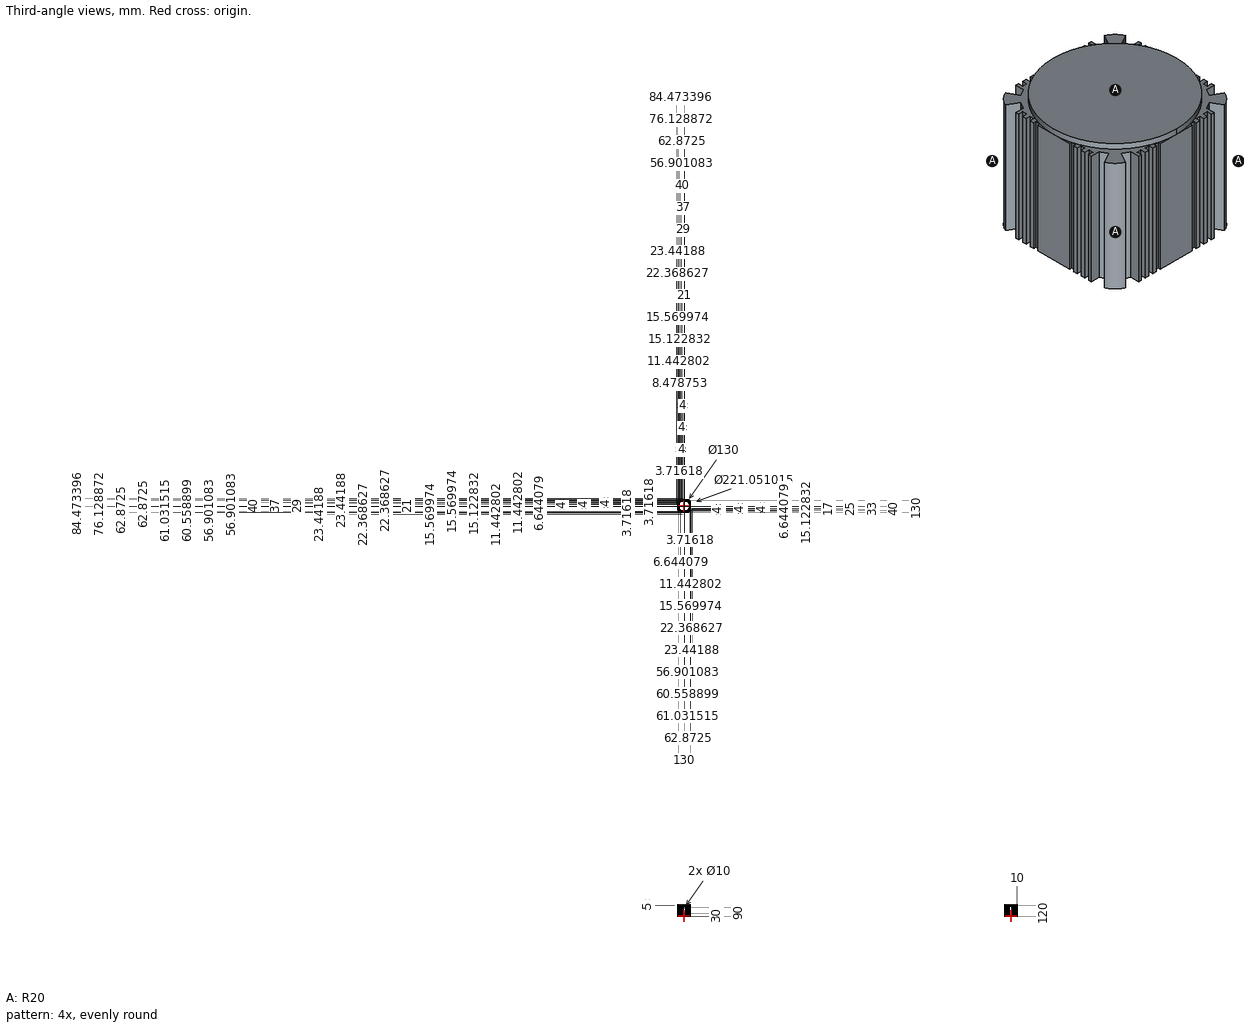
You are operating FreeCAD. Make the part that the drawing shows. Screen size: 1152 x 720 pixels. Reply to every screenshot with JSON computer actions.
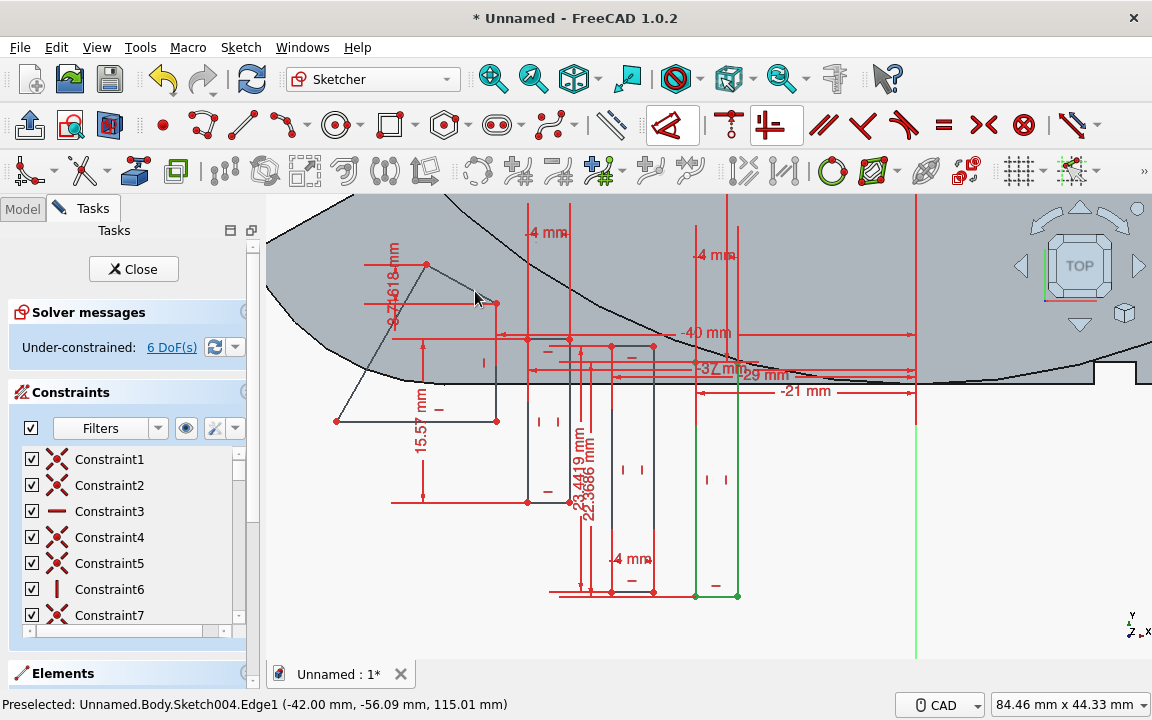
{"action": "left_click", "coordinate": [385, 422]}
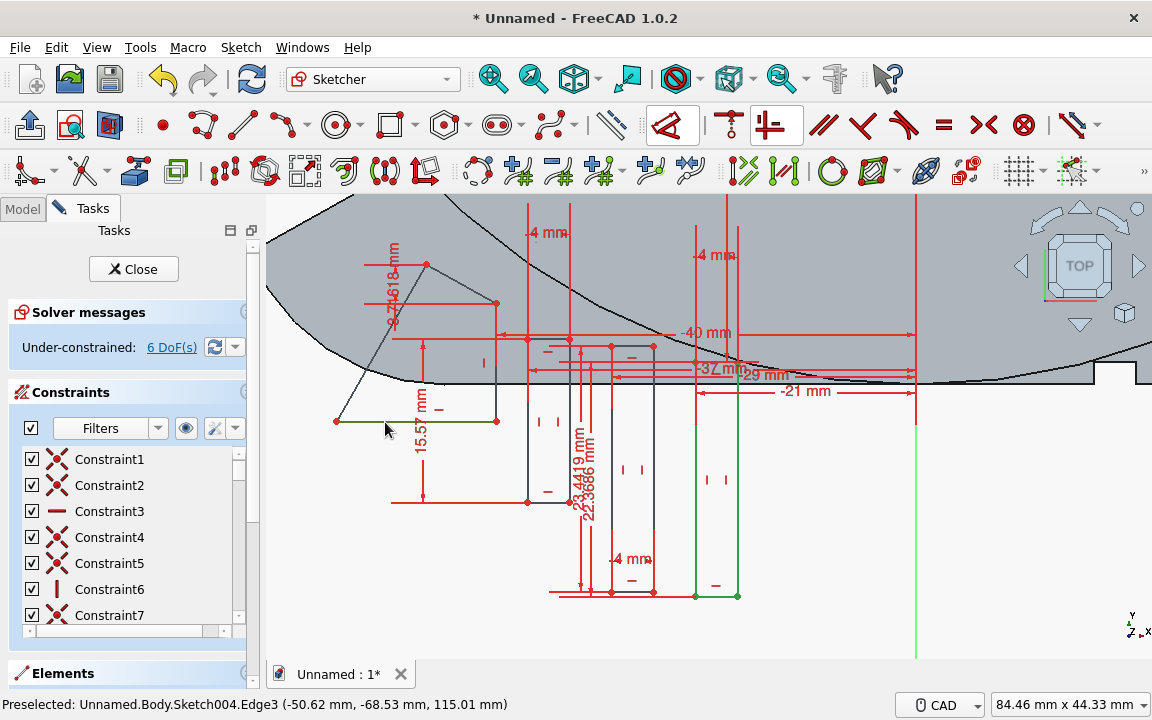
{"action": "left_click", "coordinate": [694, 126]}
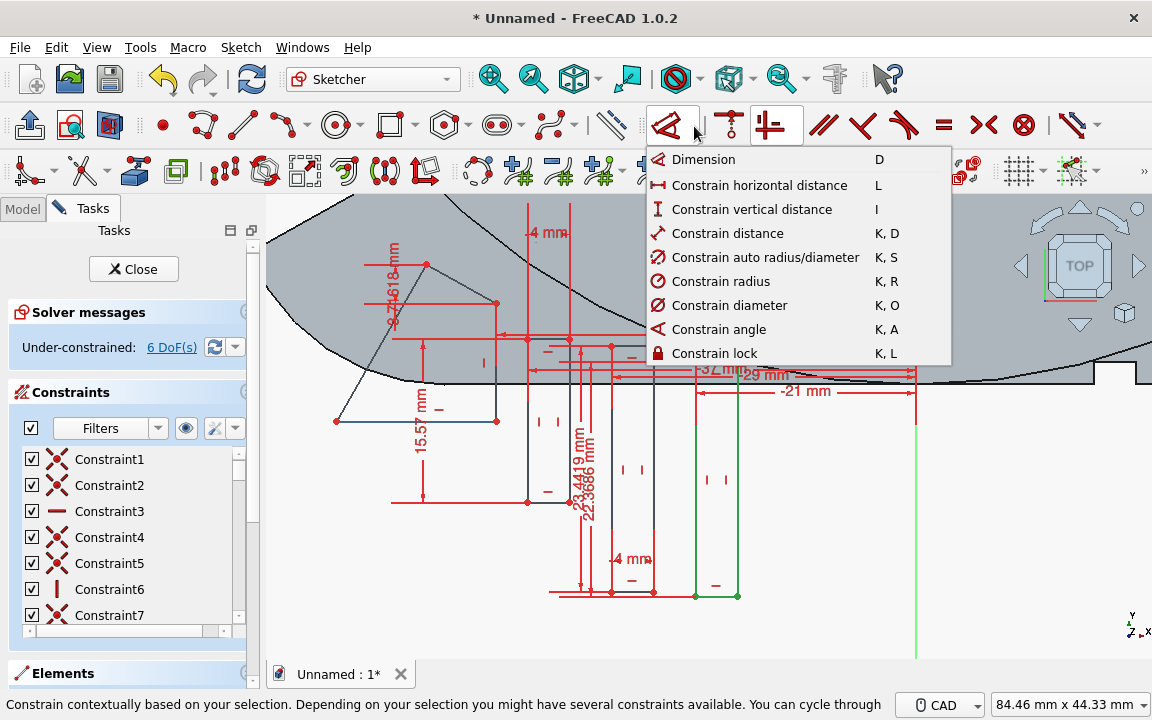
{"action": "left_click", "coordinate": [799, 185]}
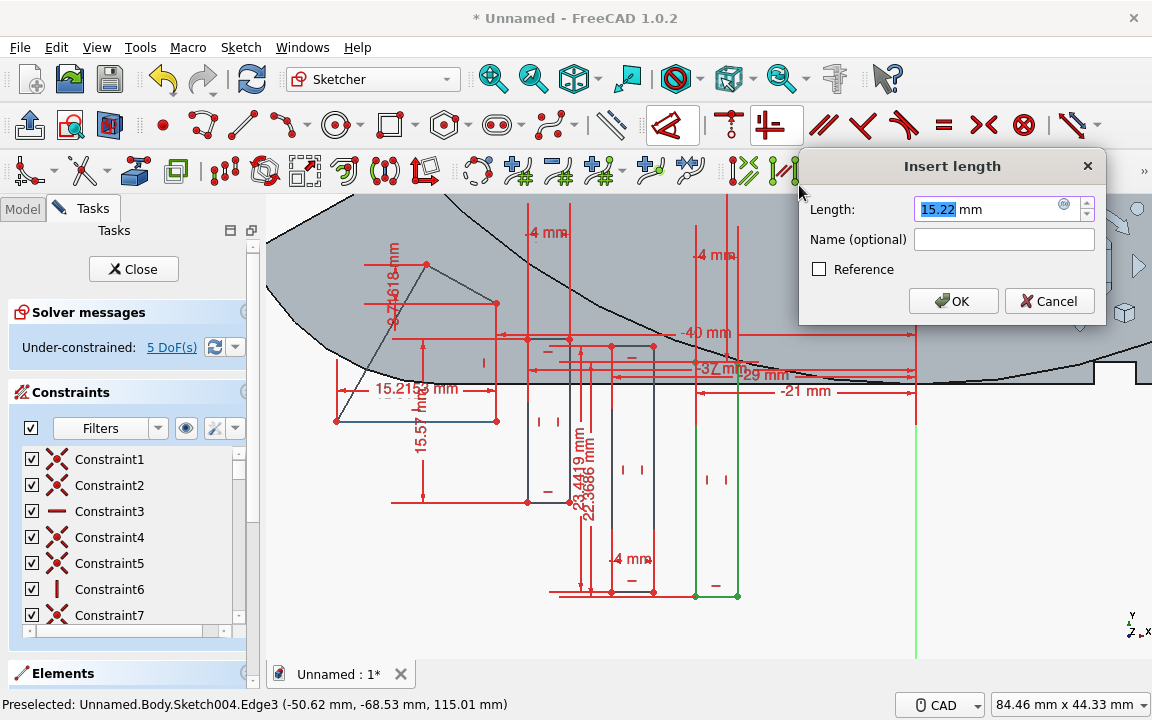
{"action": "type", "text": "15.122832"}
{"action": "key", "text": "Return"}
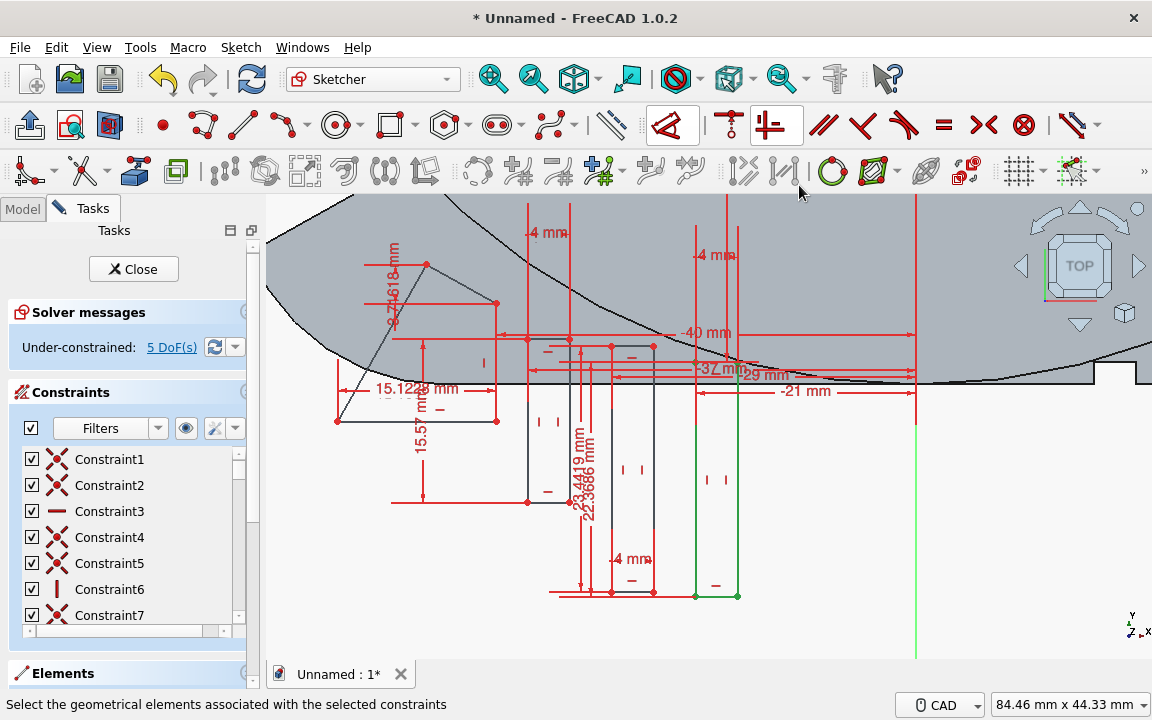
{"action": "left_click", "coordinate": [496, 386]}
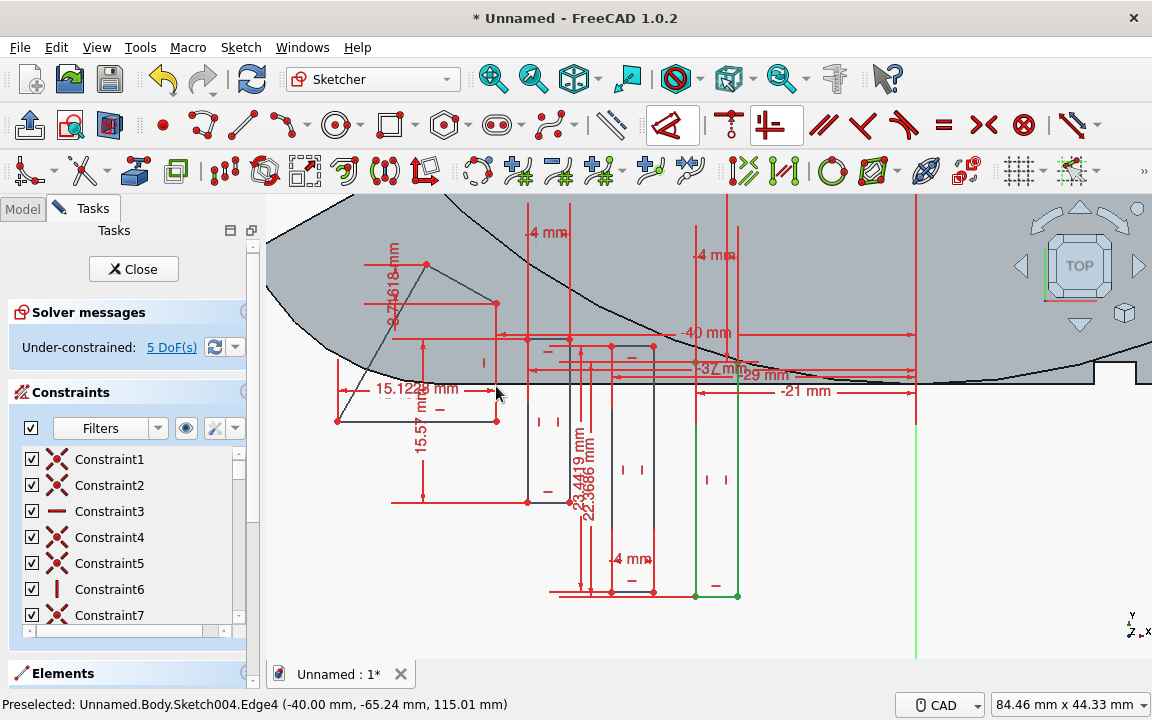
{"action": "key", "text": "i"}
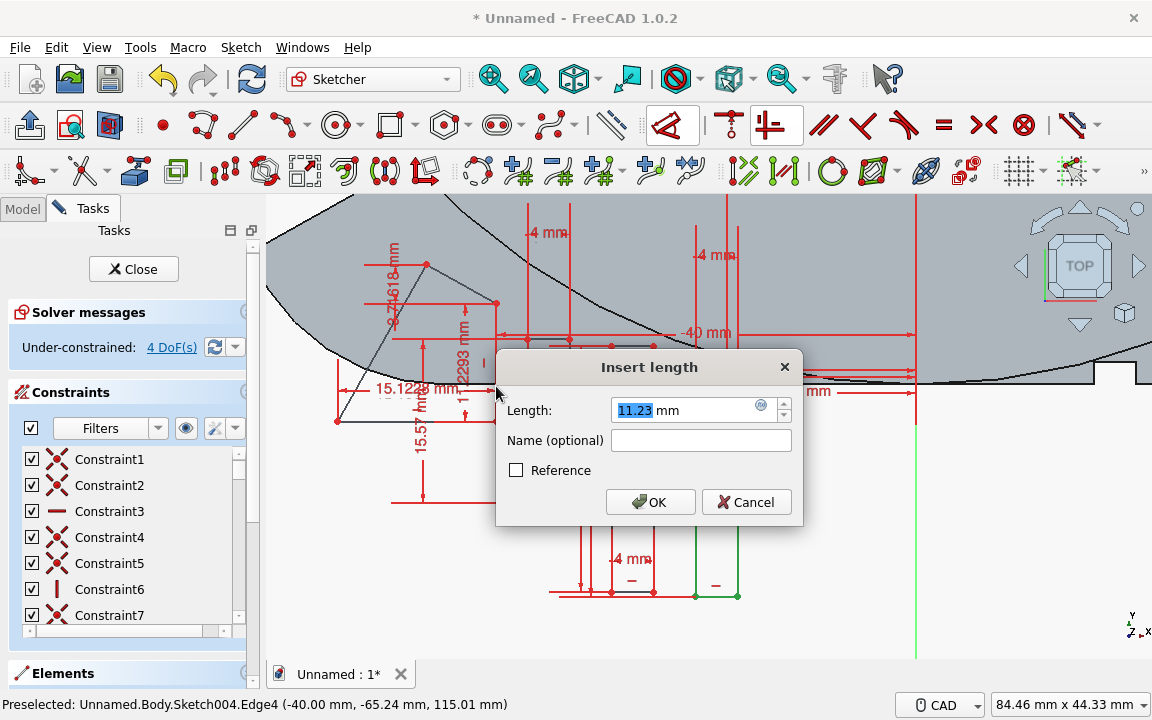
{"action": "type", "text": "11.442802"}
{"action": "key", "text": "Return"}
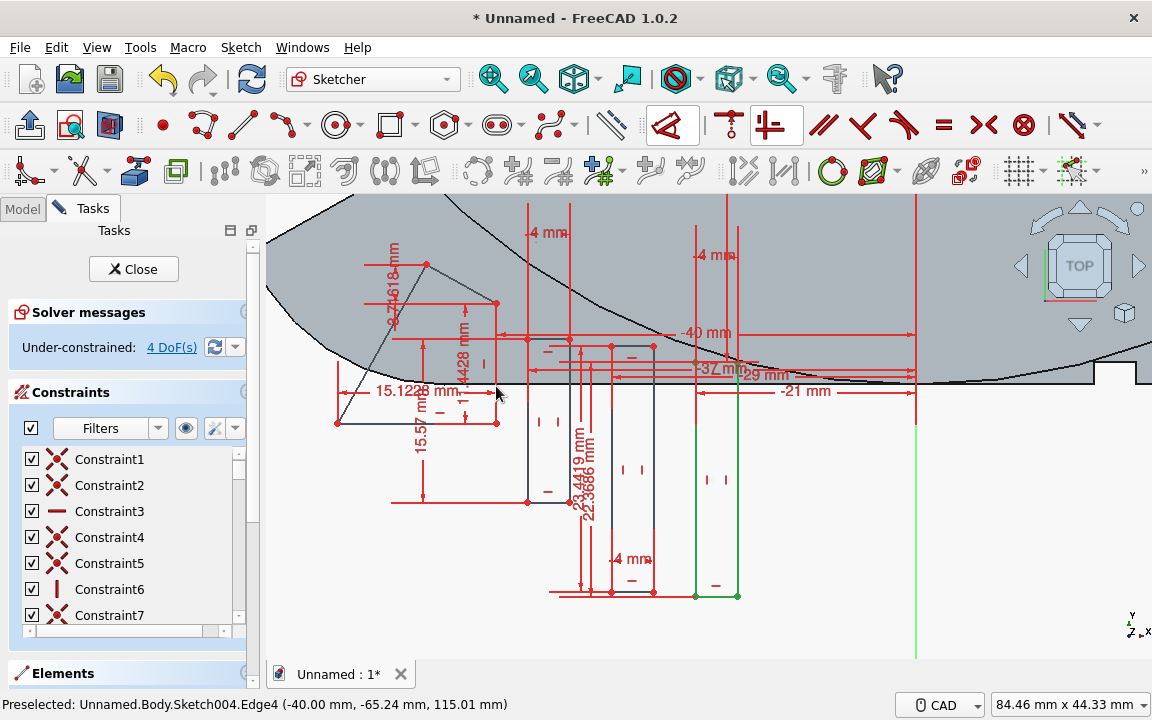
{"action": "left_click", "coordinate": [475, 292]}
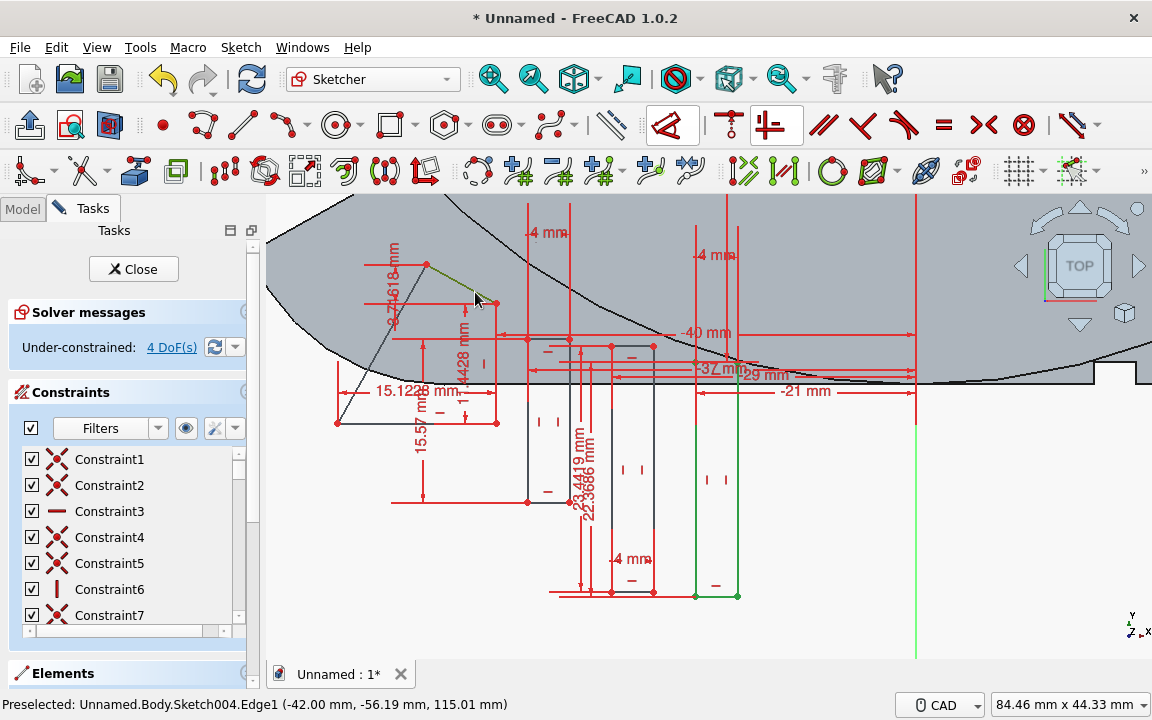
{"action": "key", "text": "l"}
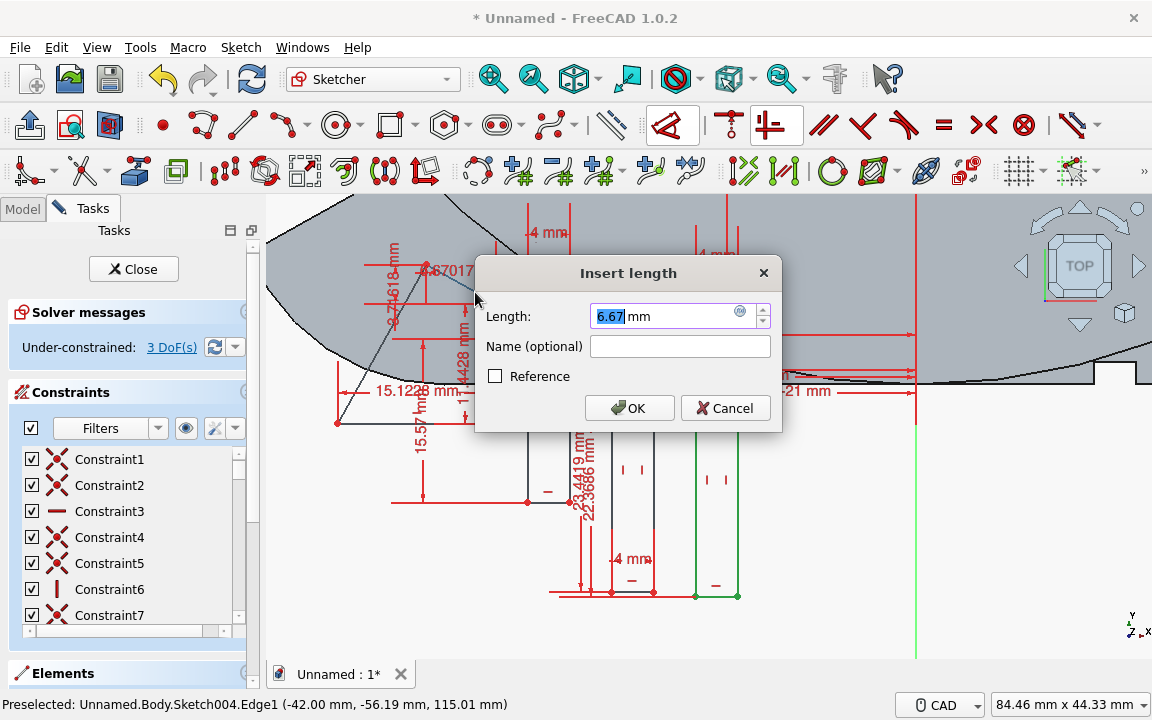
{"action": "type", "text": "6.644079"}
{"action": "key", "text": "Return"}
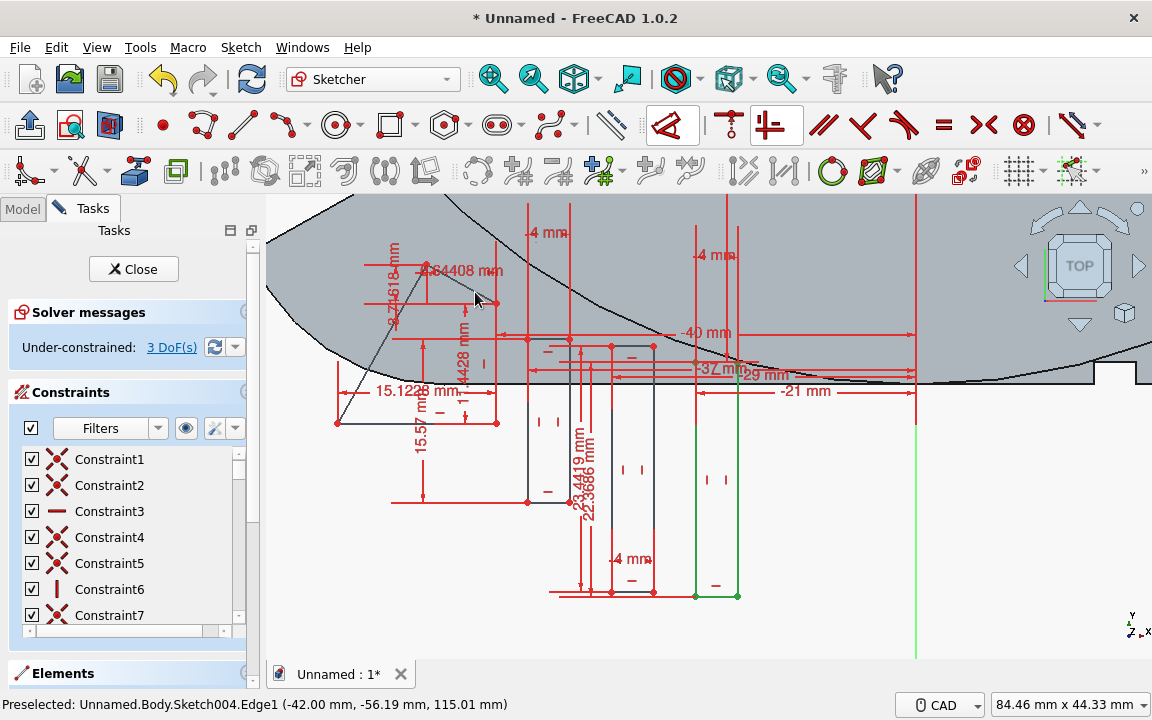
{"action": "left_click", "coordinate": [496, 304]}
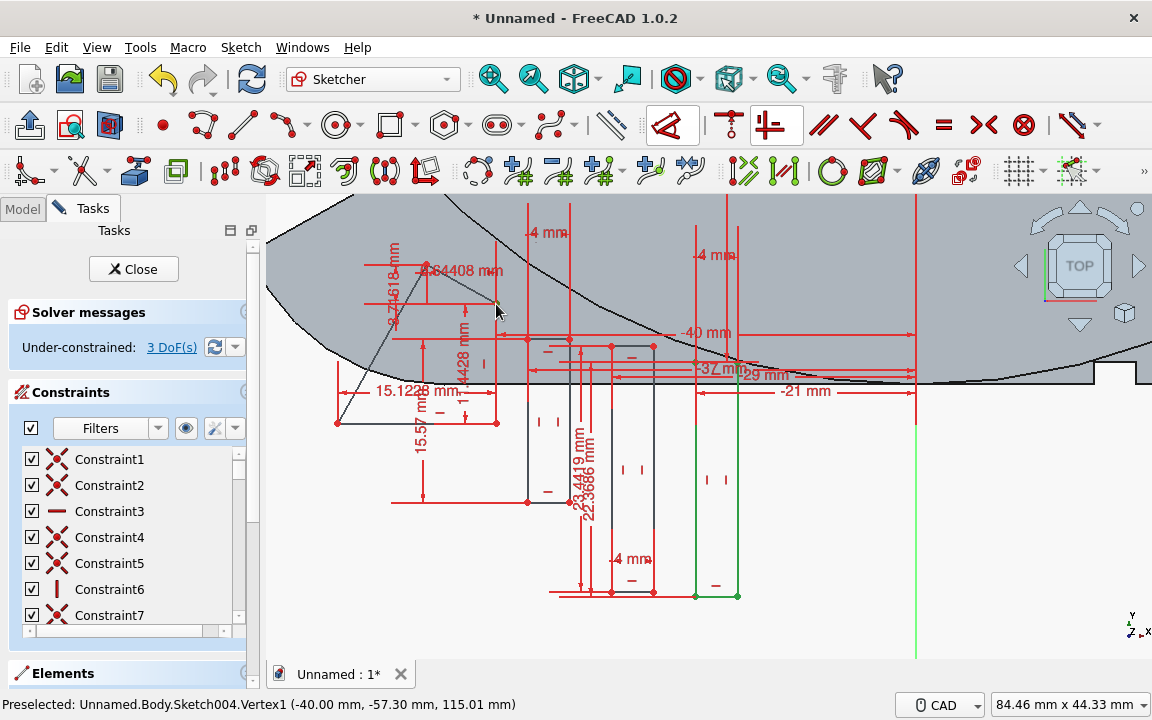
{"action": "left_click", "coordinate": [694, 126]}